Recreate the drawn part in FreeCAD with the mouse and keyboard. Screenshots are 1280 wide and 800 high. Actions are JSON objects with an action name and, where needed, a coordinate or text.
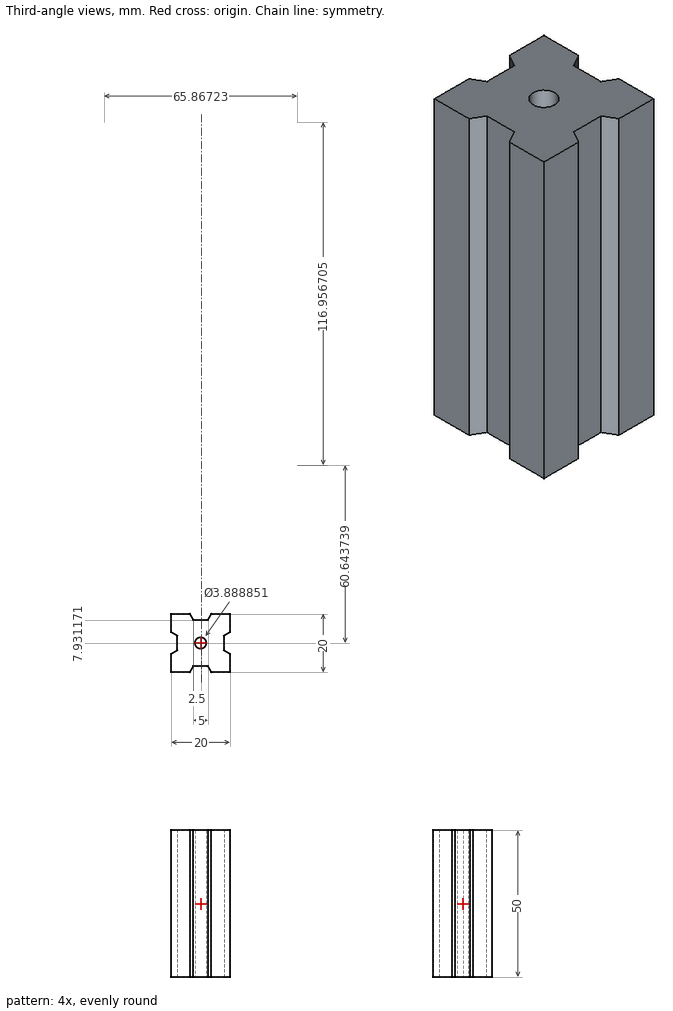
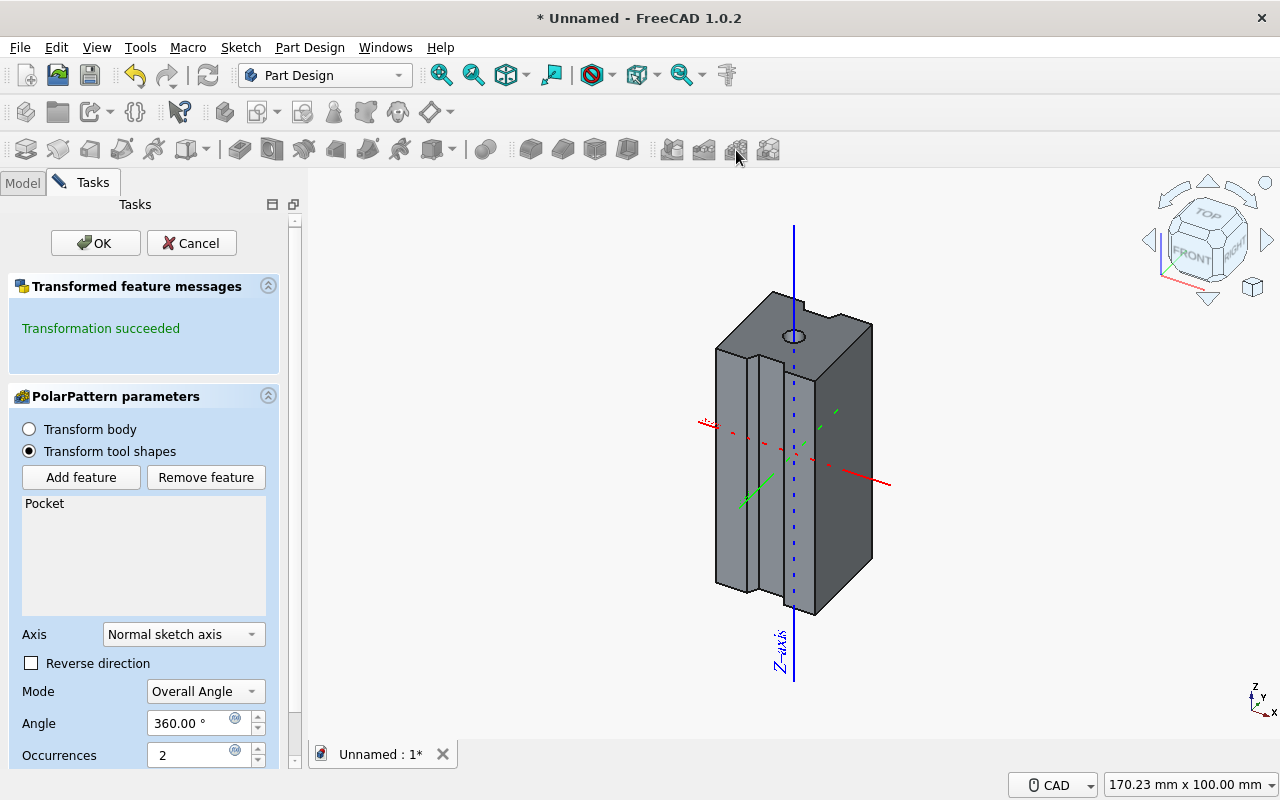
{"action": "left_click", "coordinate": [184, 634]}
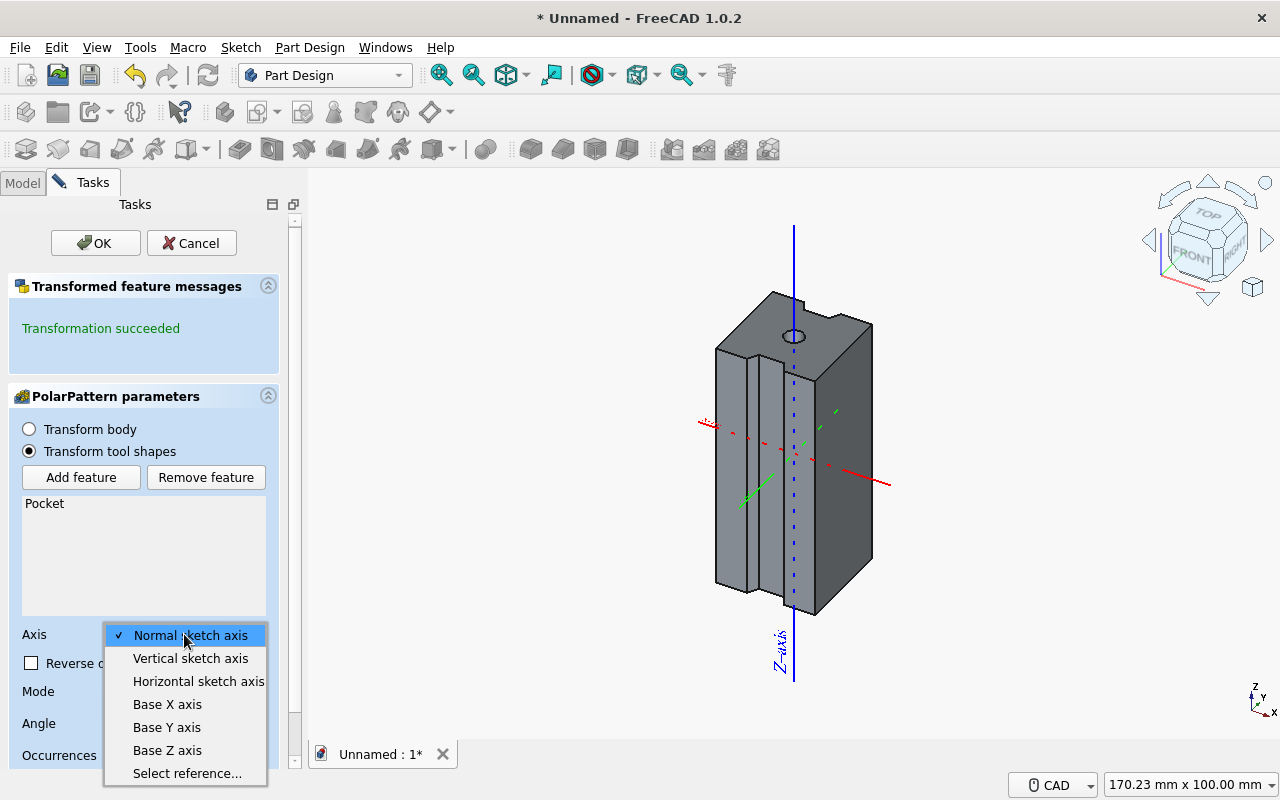
{"action": "left_click", "coordinate": [184, 750]}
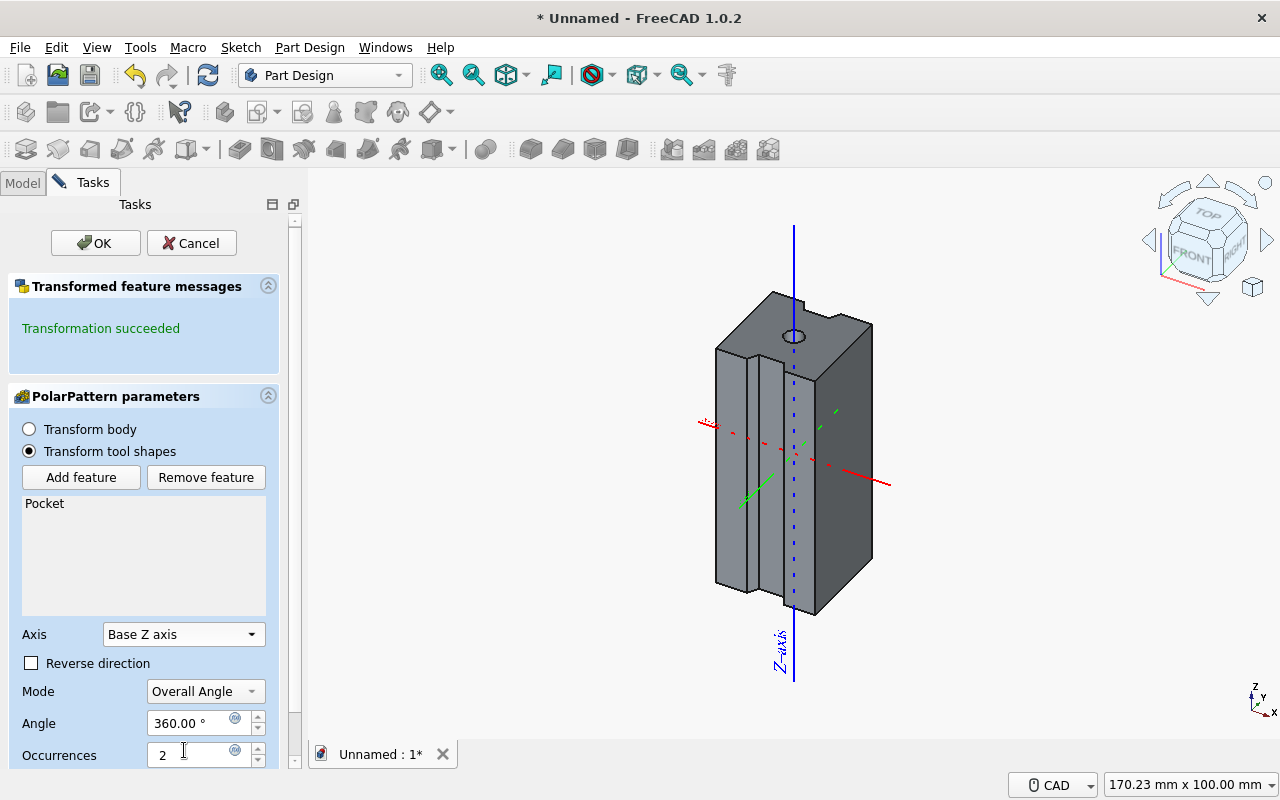
{"action": "triple_click", "coordinate": [198, 755]}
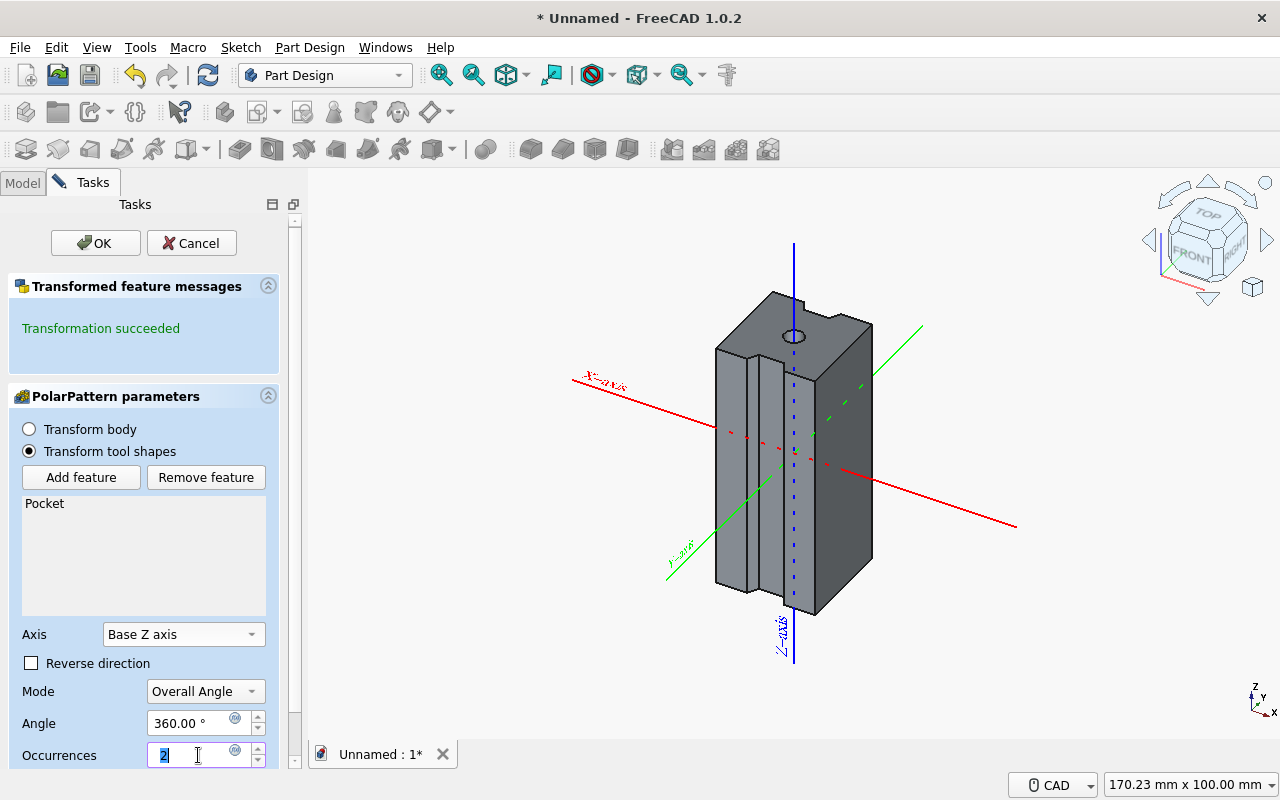
{"action": "type", "text": "4"}
{"action": "key", "text": "Tab"}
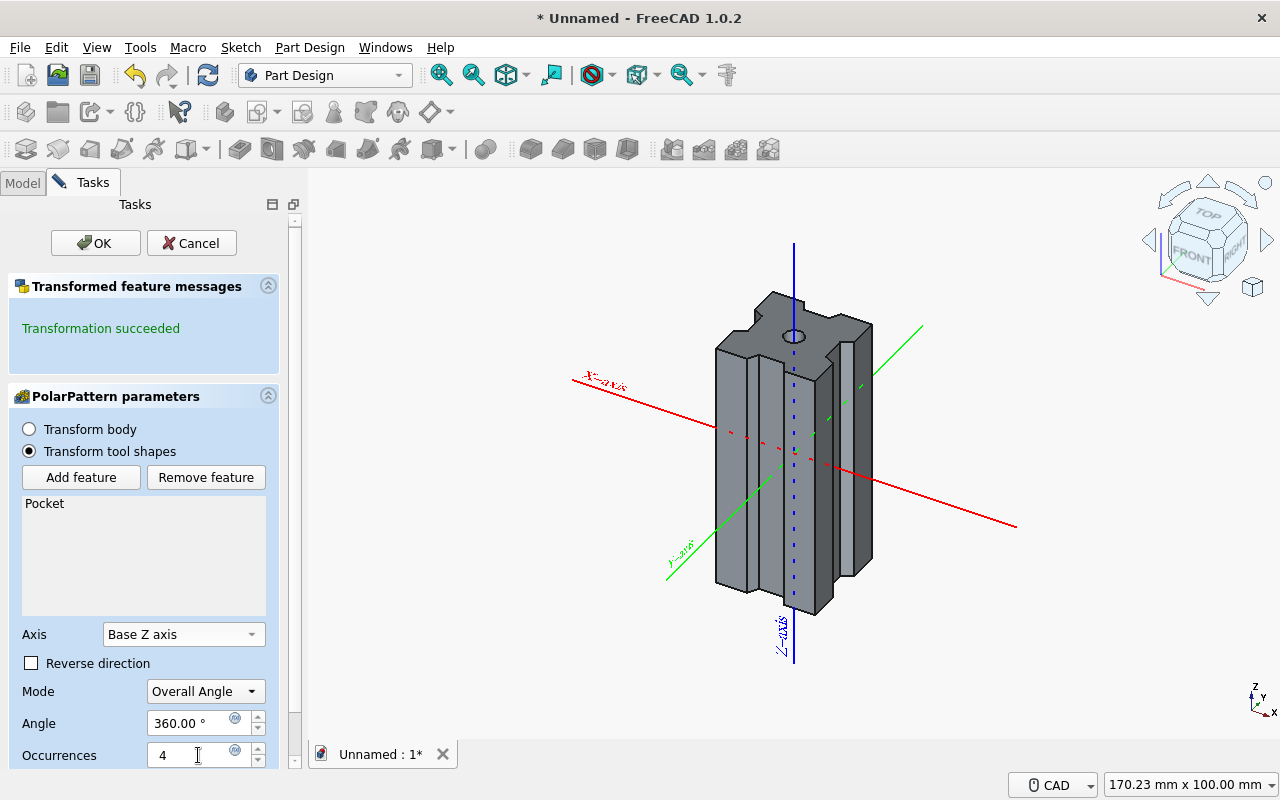
{"action": "left_click", "coordinate": [96, 243]}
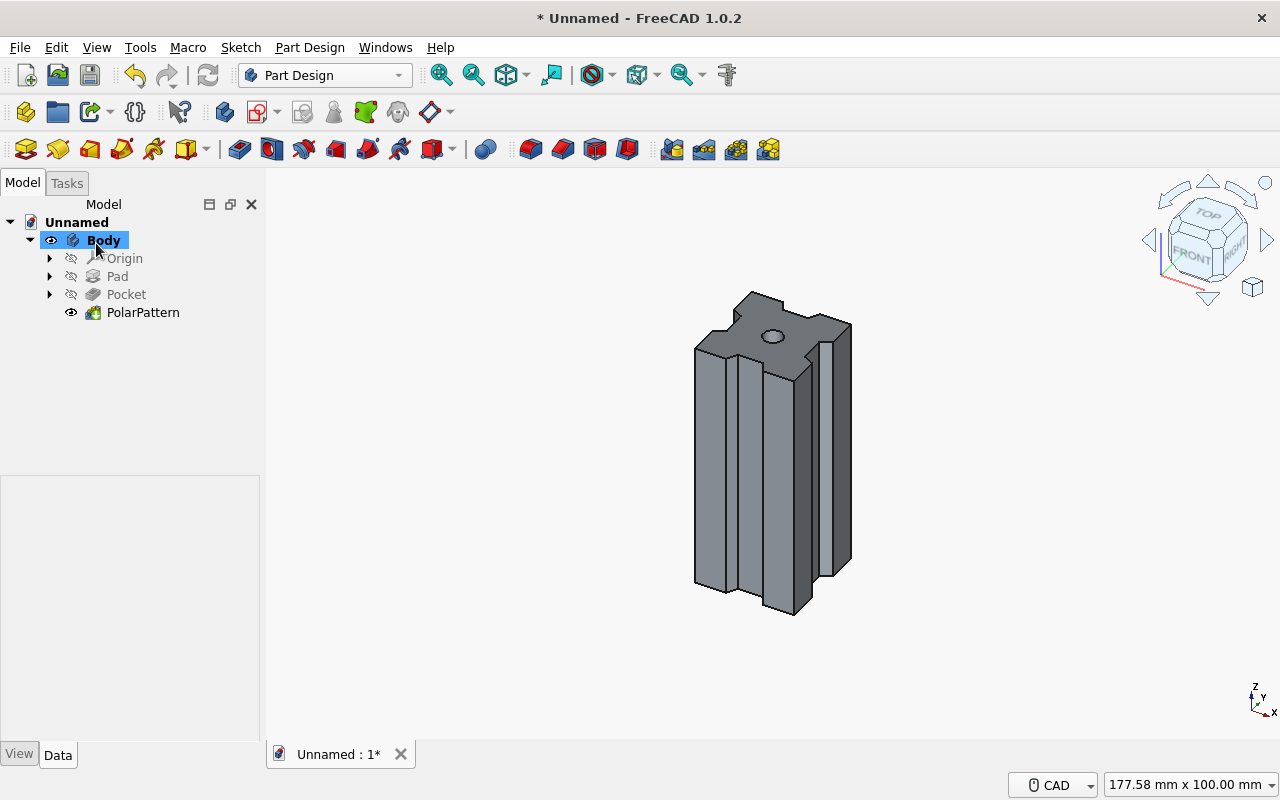
{"action": "key", "text": "0"}